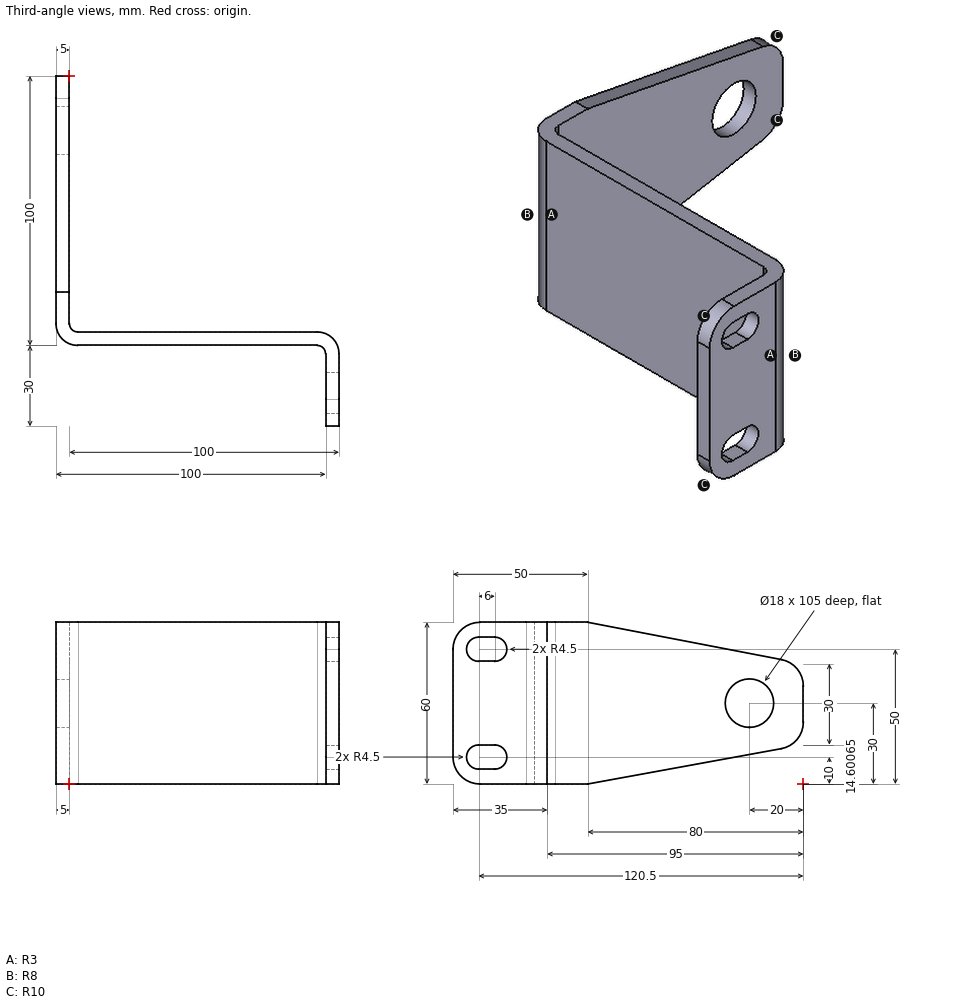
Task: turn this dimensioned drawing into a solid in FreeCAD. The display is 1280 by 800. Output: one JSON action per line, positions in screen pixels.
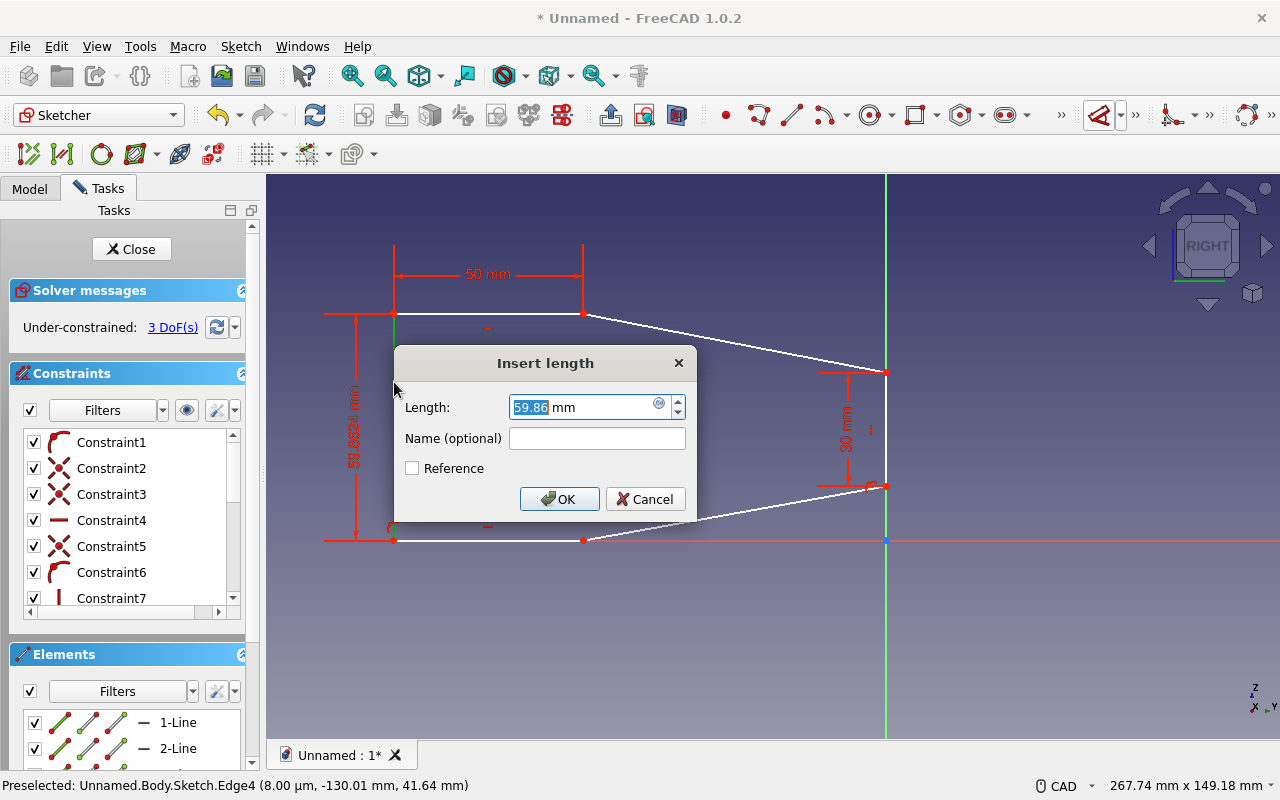
{"action": "type", "text": "60"}
{"action": "key", "text": "Return"}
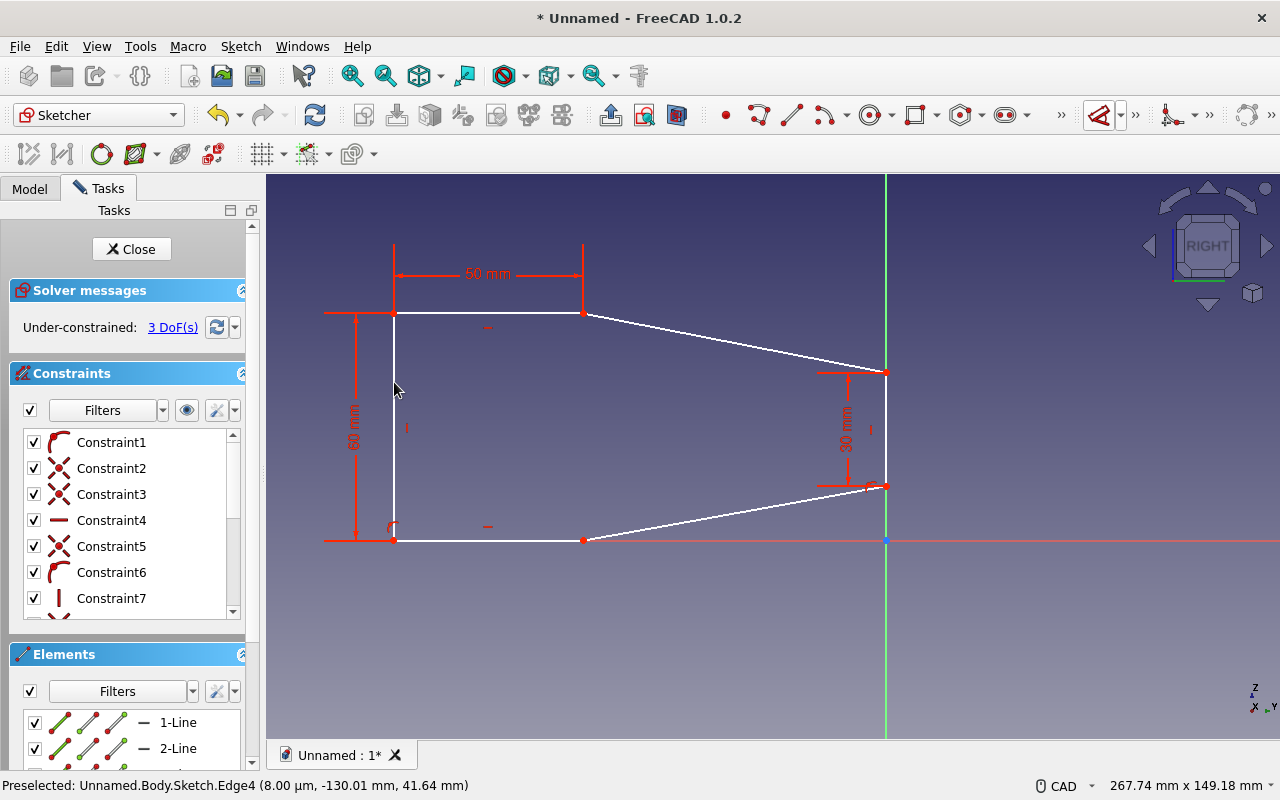
{"action": "left_click", "coordinate": [450, 541]}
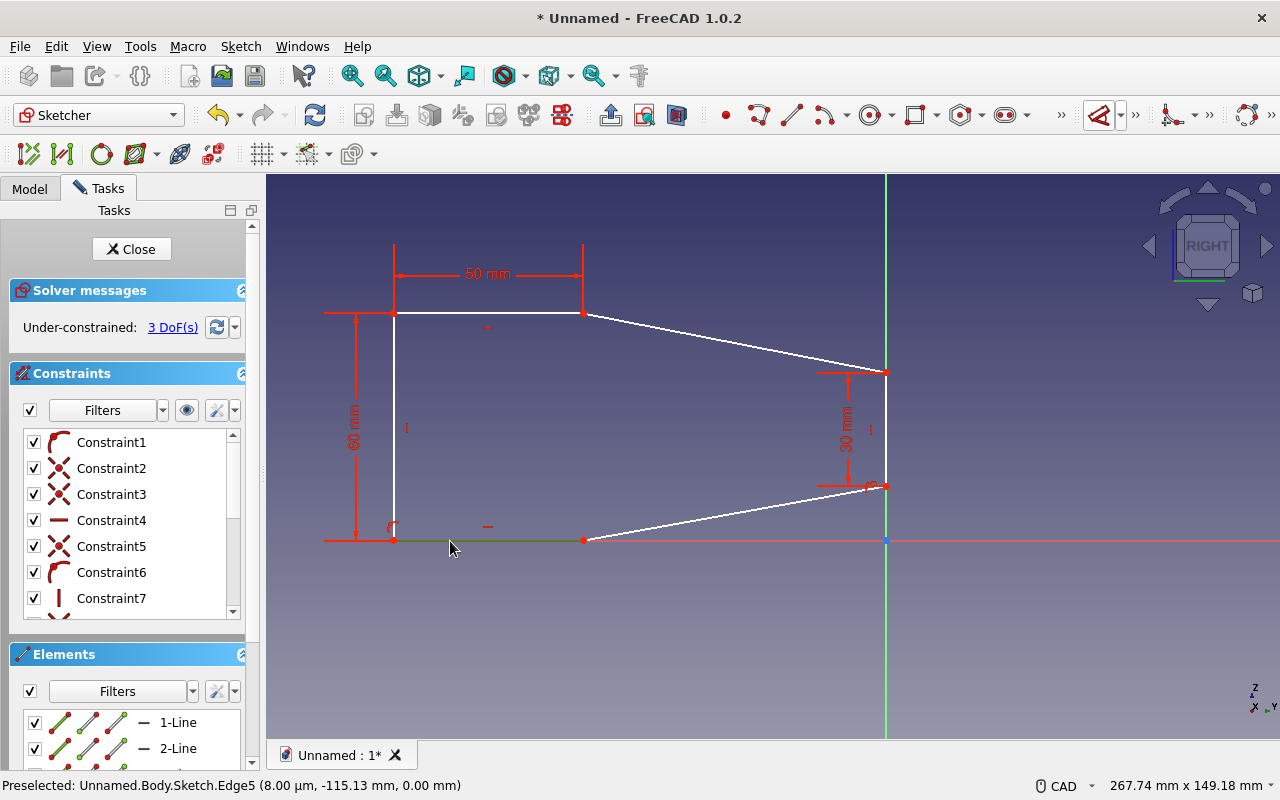
{"action": "key", "text": "l"}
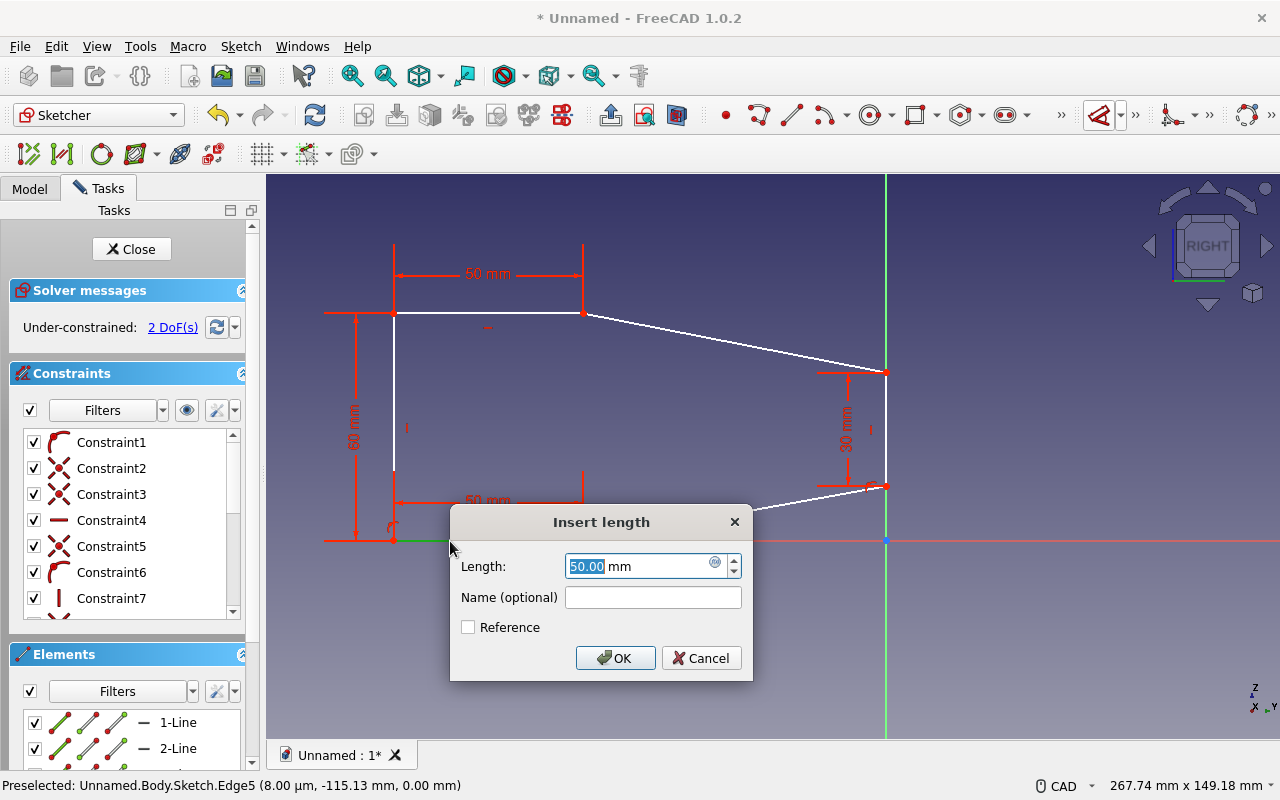
{"action": "type", "text": "50"}
{"action": "key", "text": "Return"}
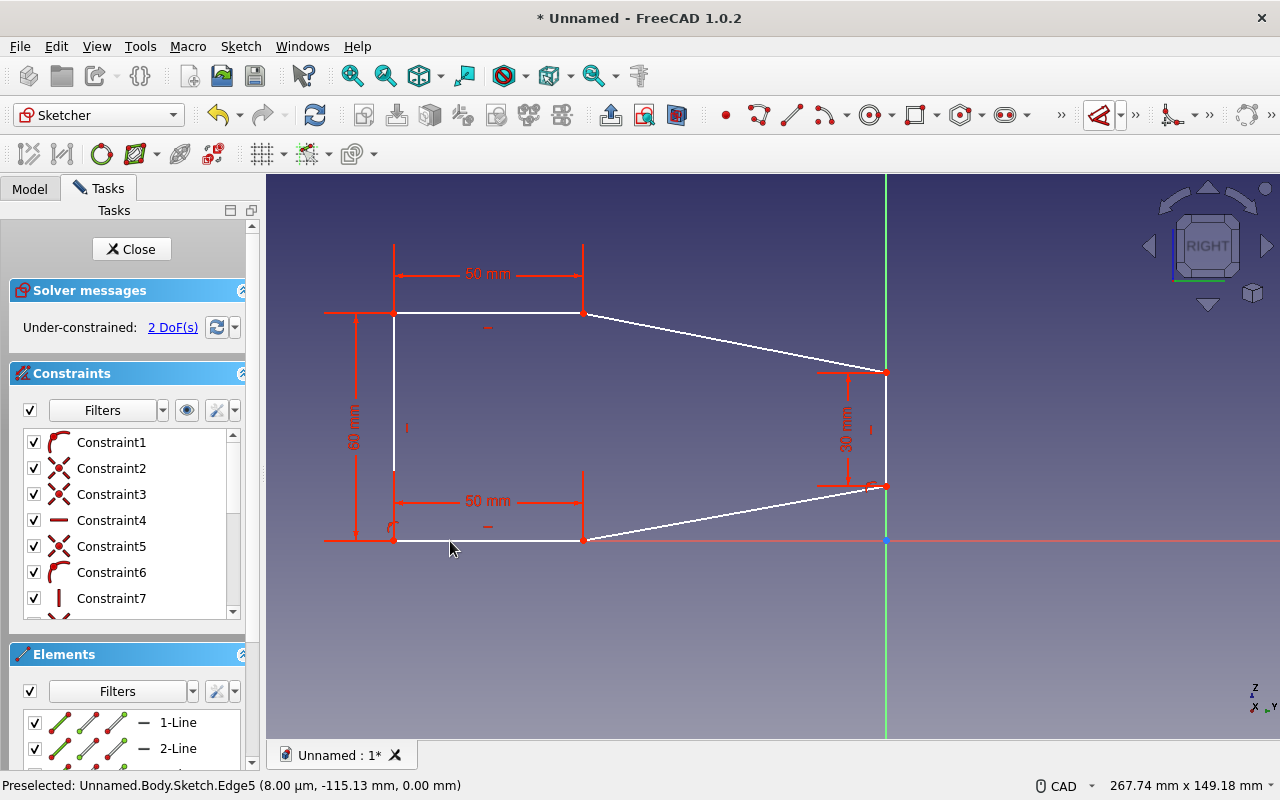
{"action": "left_click", "coordinate": [583, 313]}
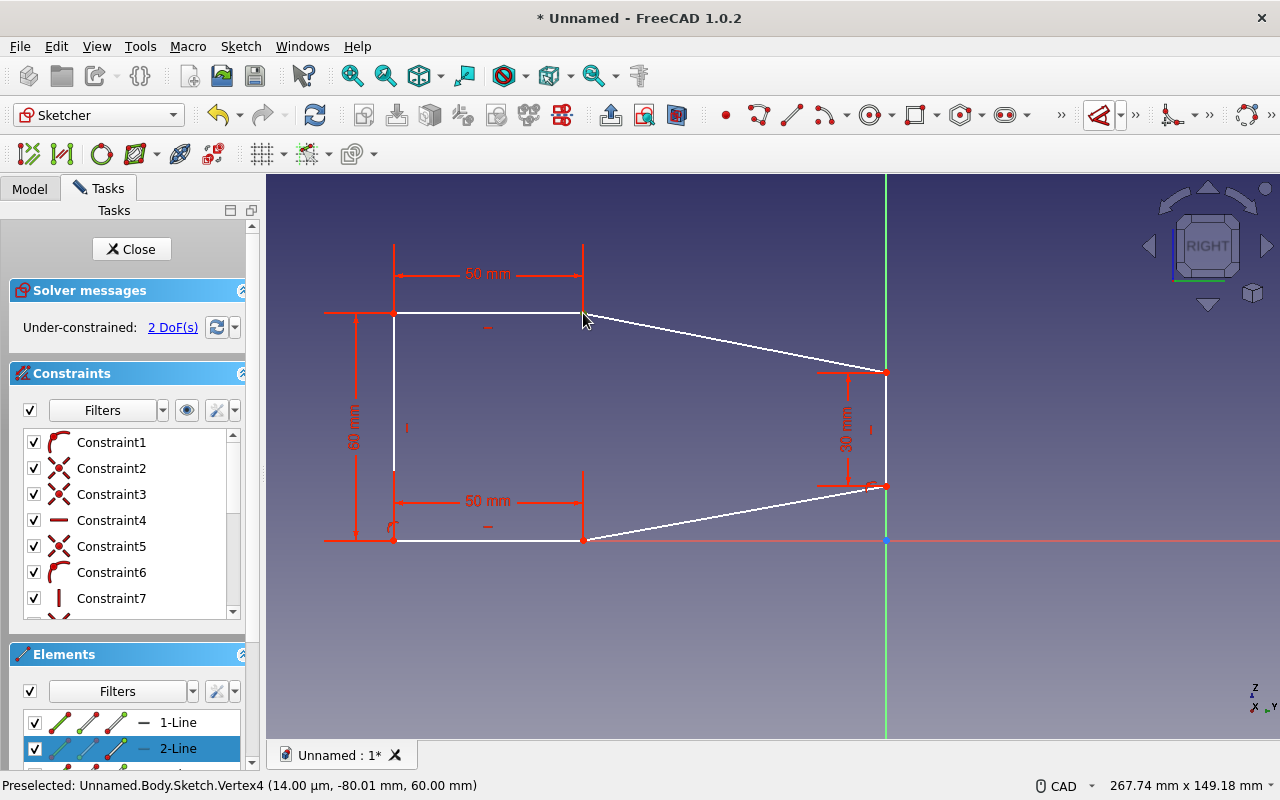
{"action": "left_click", "coordinate": [1120, 116]}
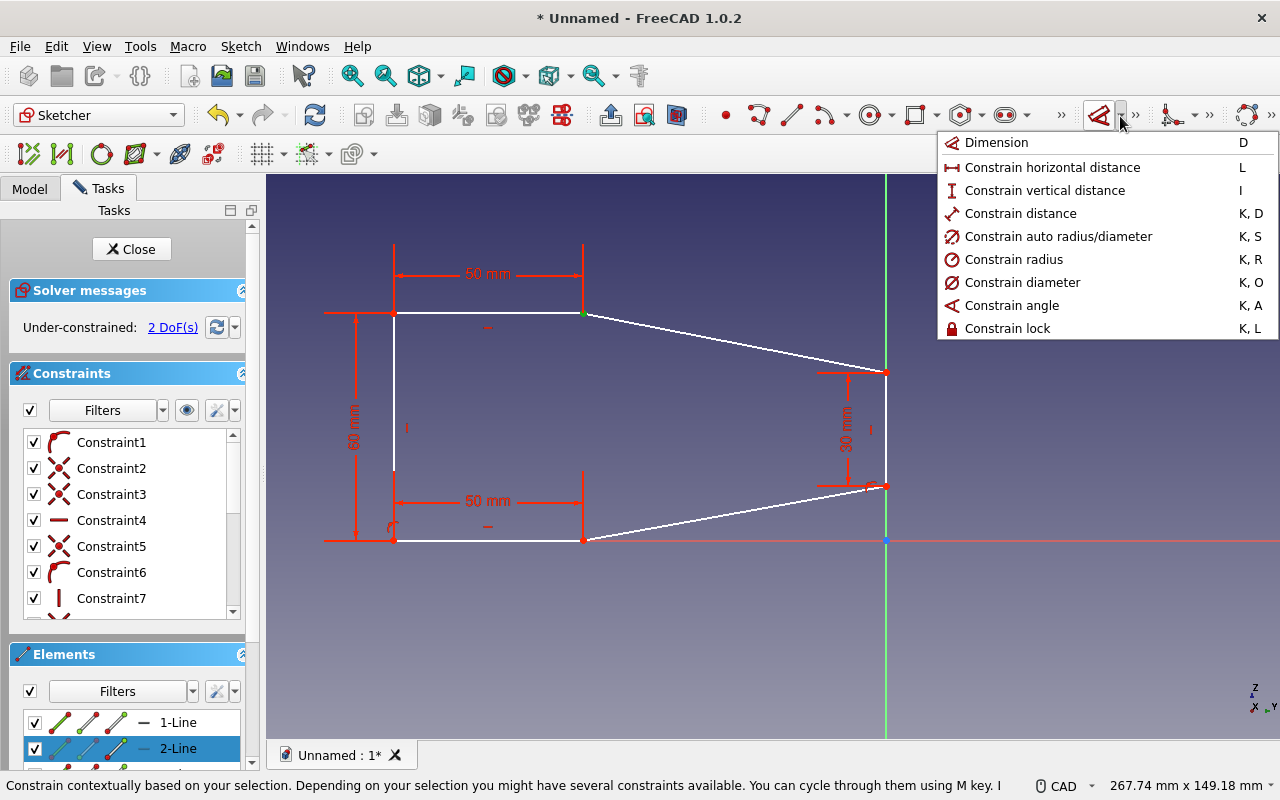
{"action": "left_click", "coordinate": [1108, 168]}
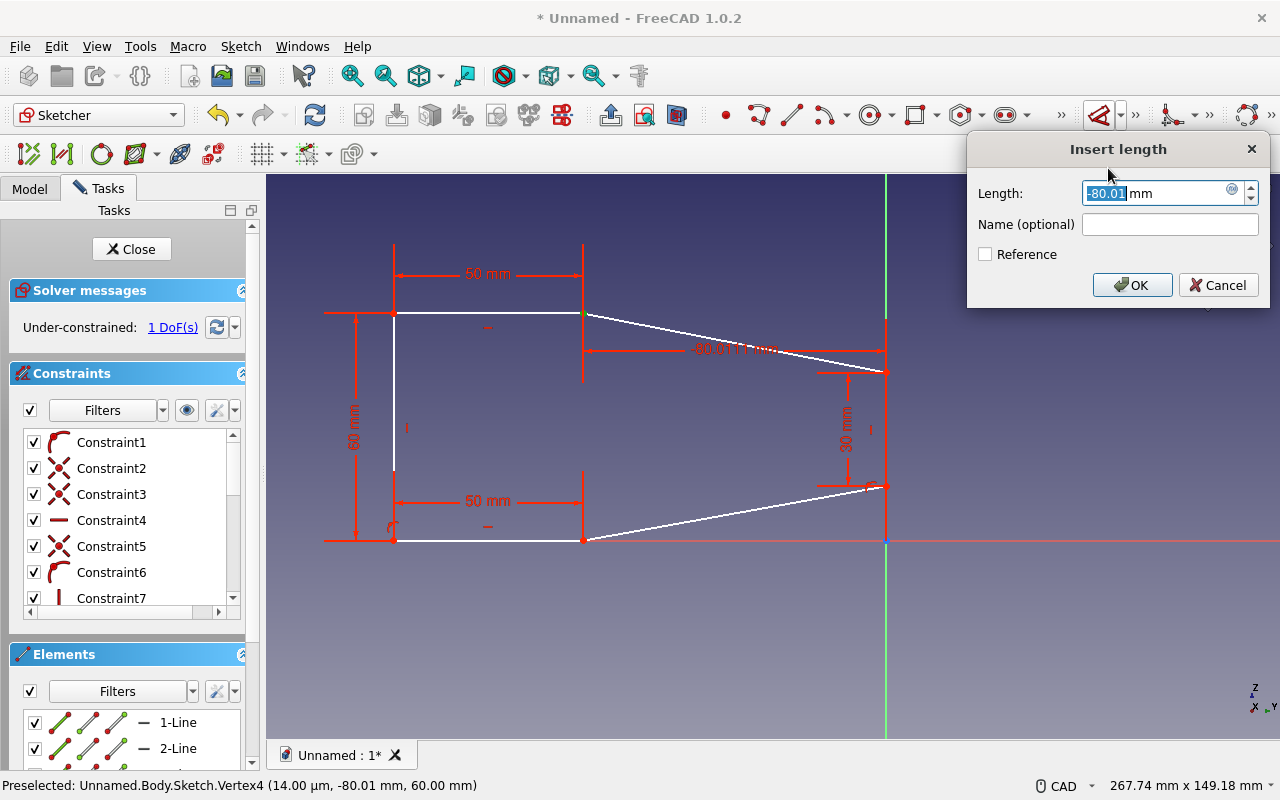
{"action": "type", "text": "-80"}
{"action": "key", "text": "Return"}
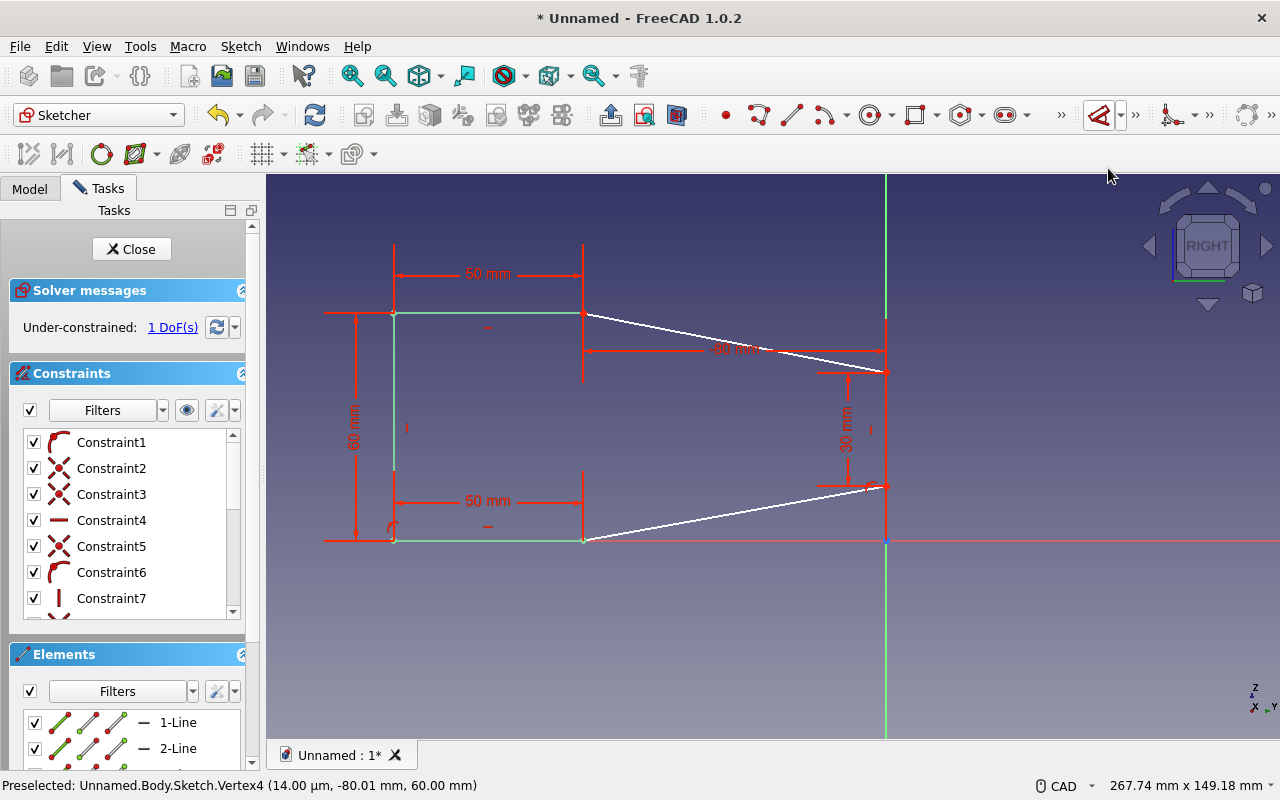
{"action": "left_click", "coordinate": [886, 486]}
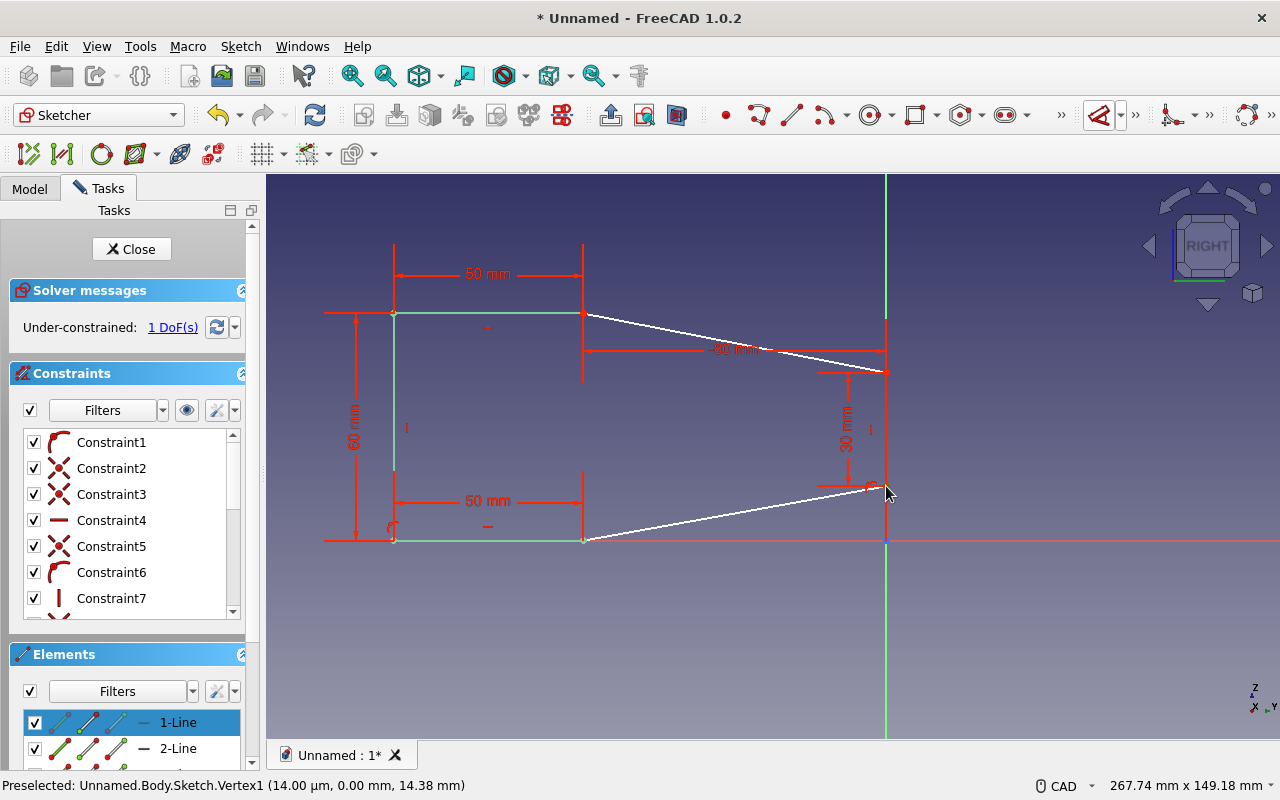
{"action": "key", "text": "i"}